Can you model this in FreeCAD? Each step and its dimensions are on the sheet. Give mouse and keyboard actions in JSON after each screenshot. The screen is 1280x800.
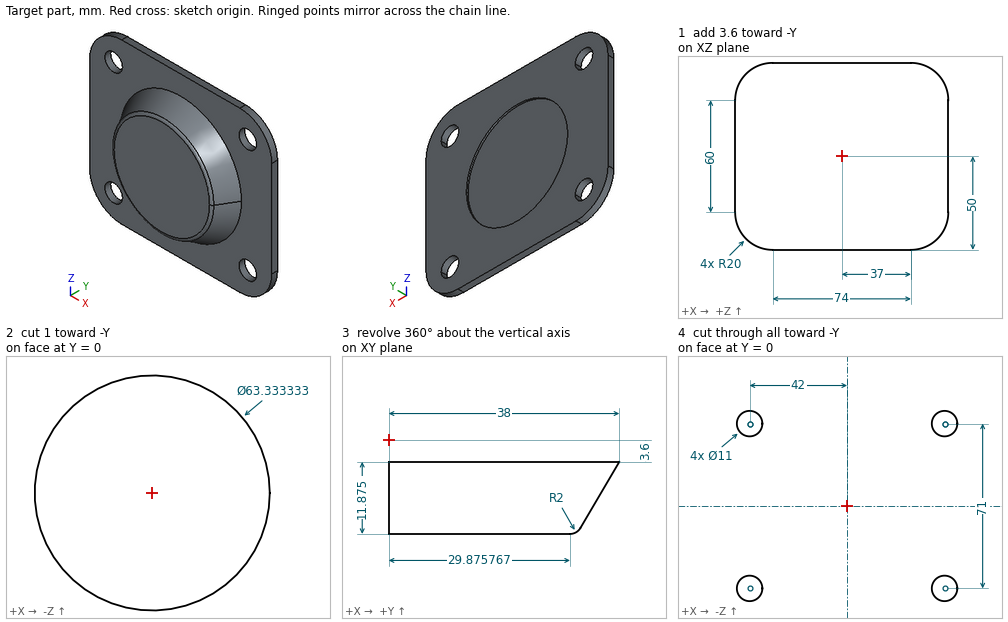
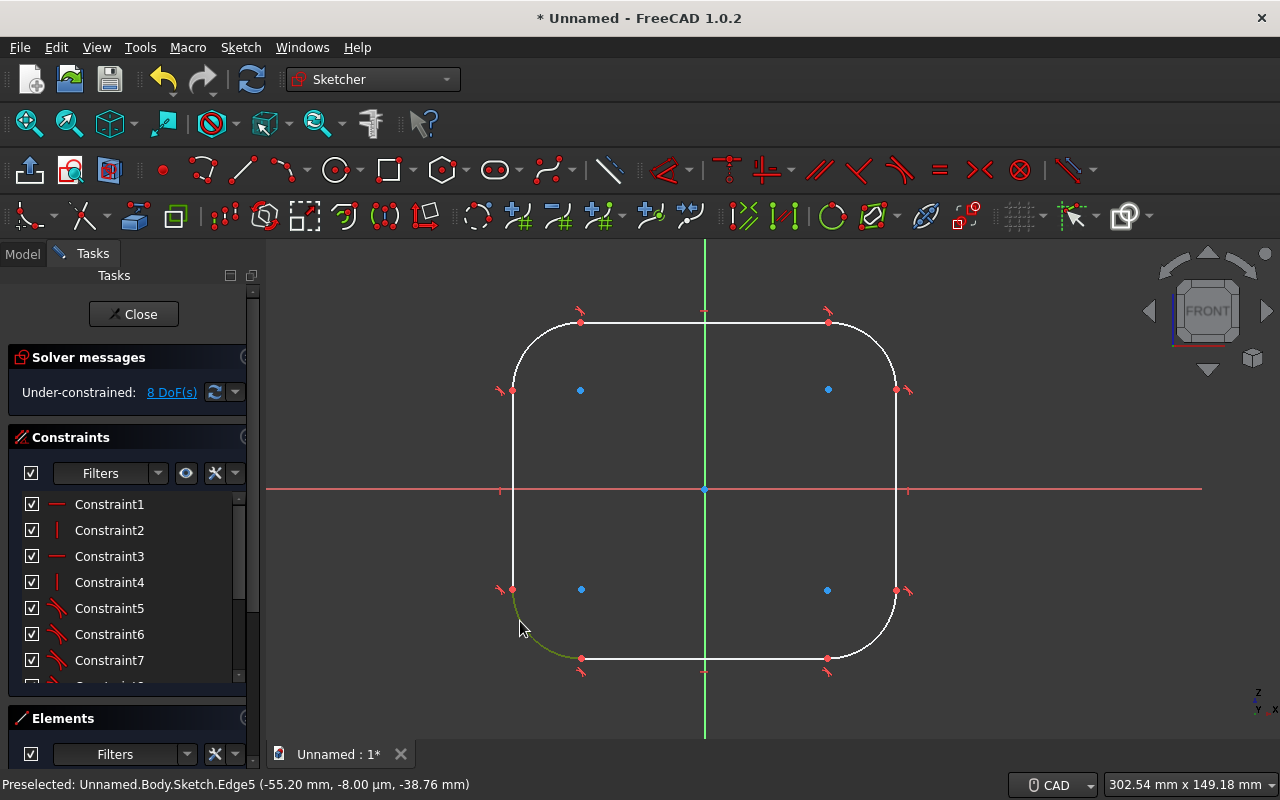
{"action": "left_click", "coordinate": [550, 330]}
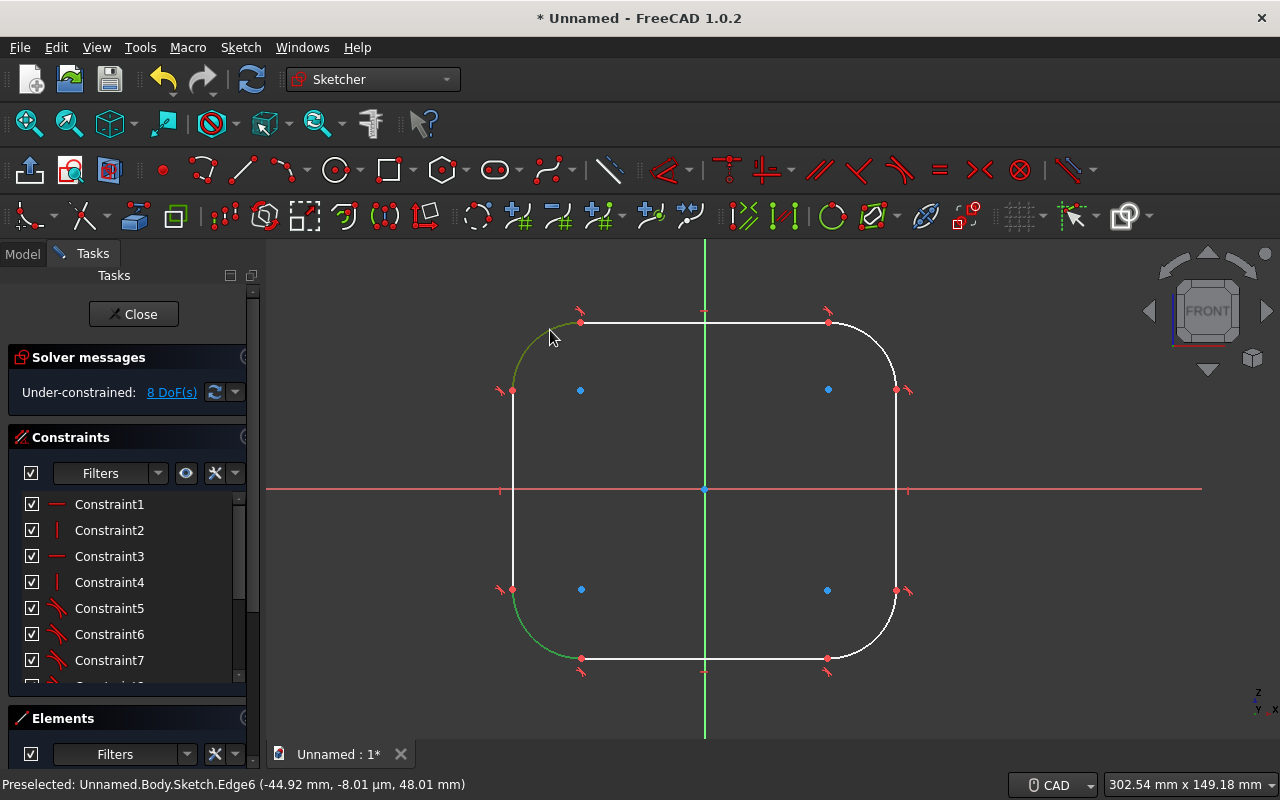
{"action": "left_click", "coordinate": [889, 359]}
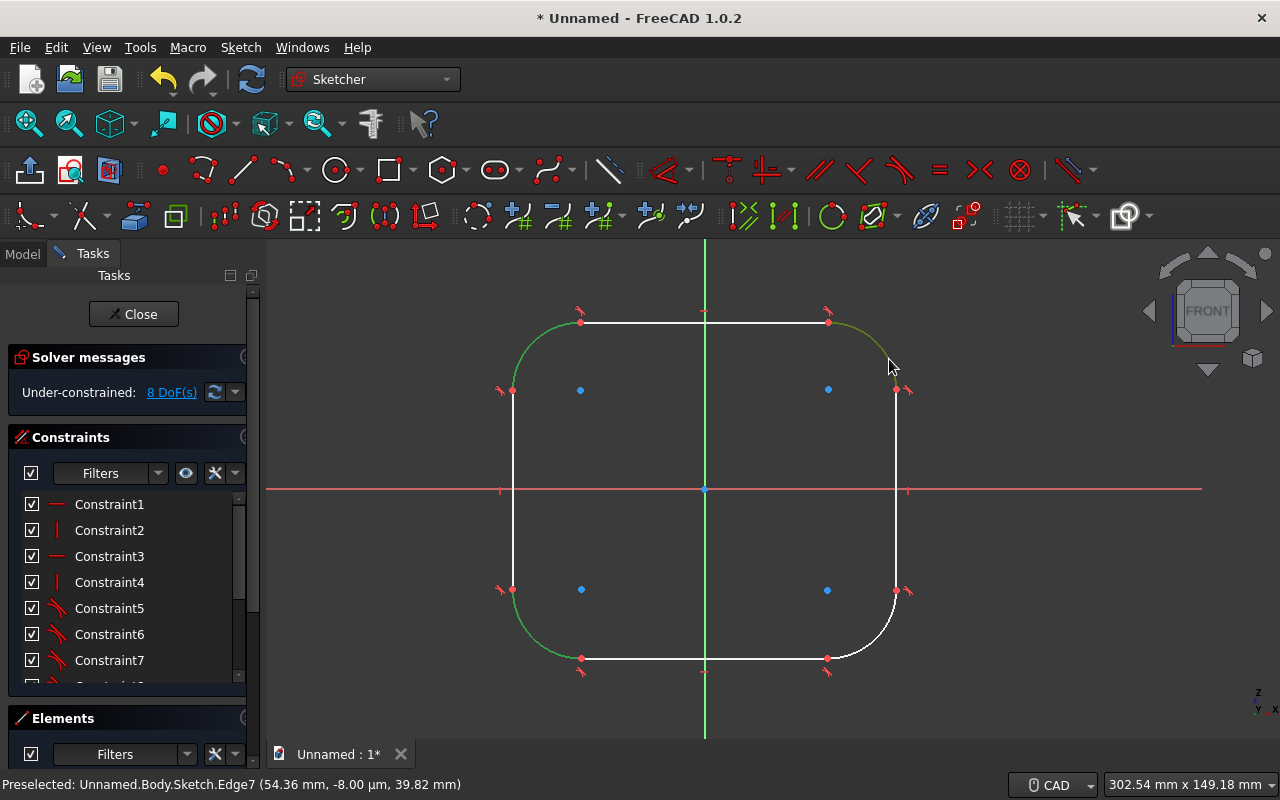
{"action": "left_click", "coordinate": [859, 651]}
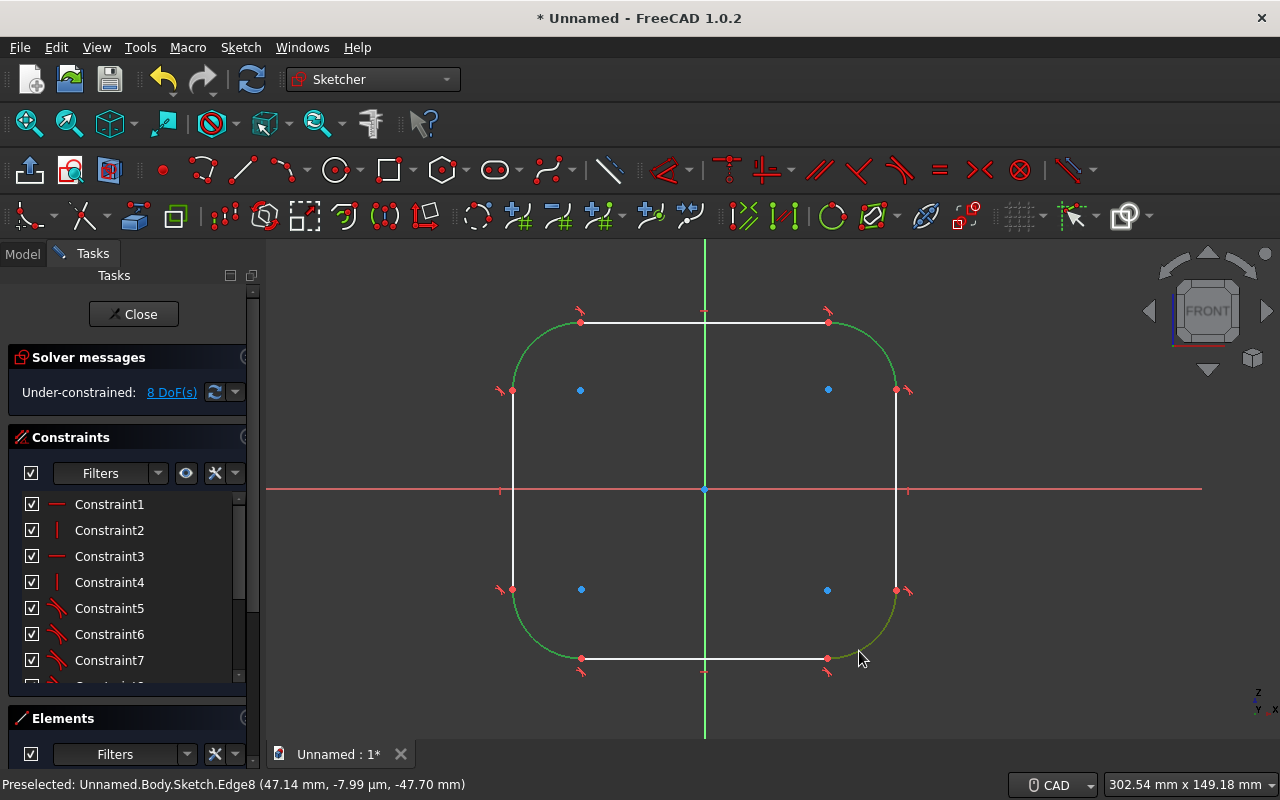
{"action": "left_click", "coordinate": [940, 170]}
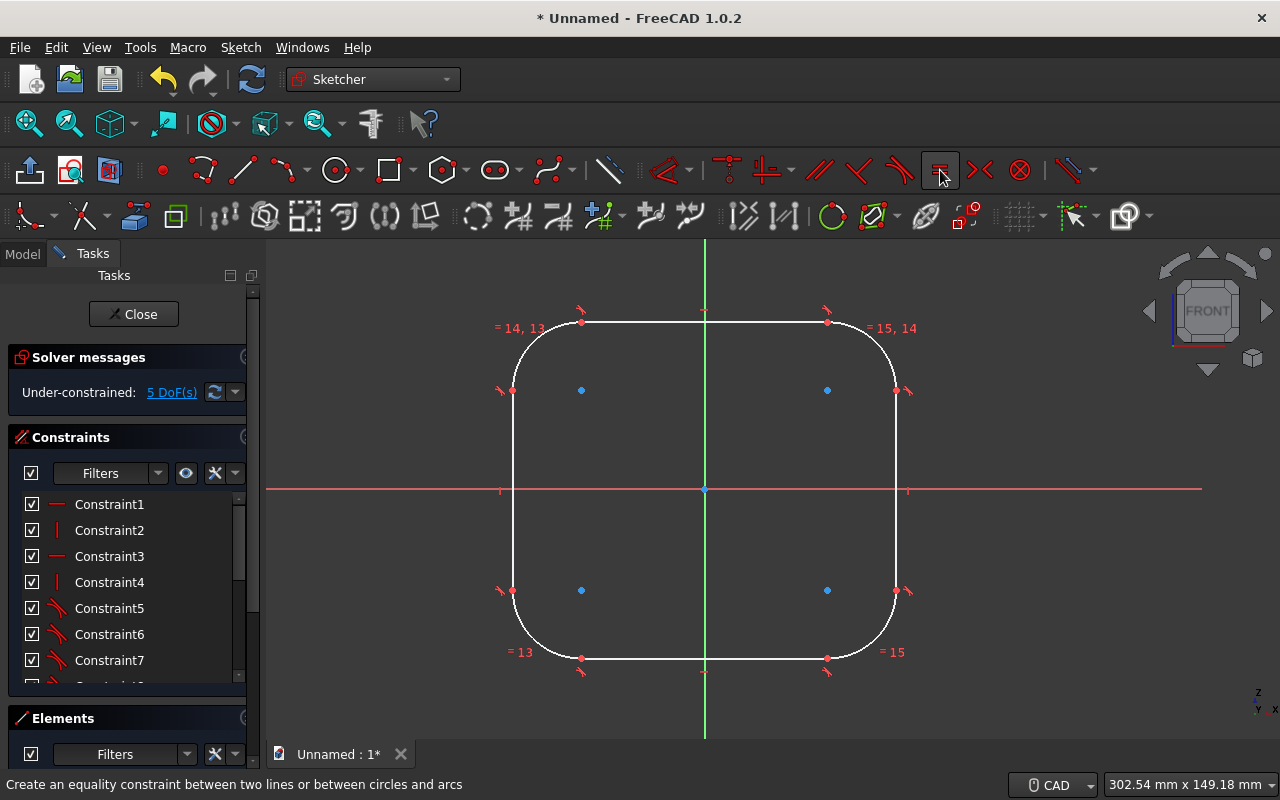
{"action": "left_click", "coordinate": [664, 170]}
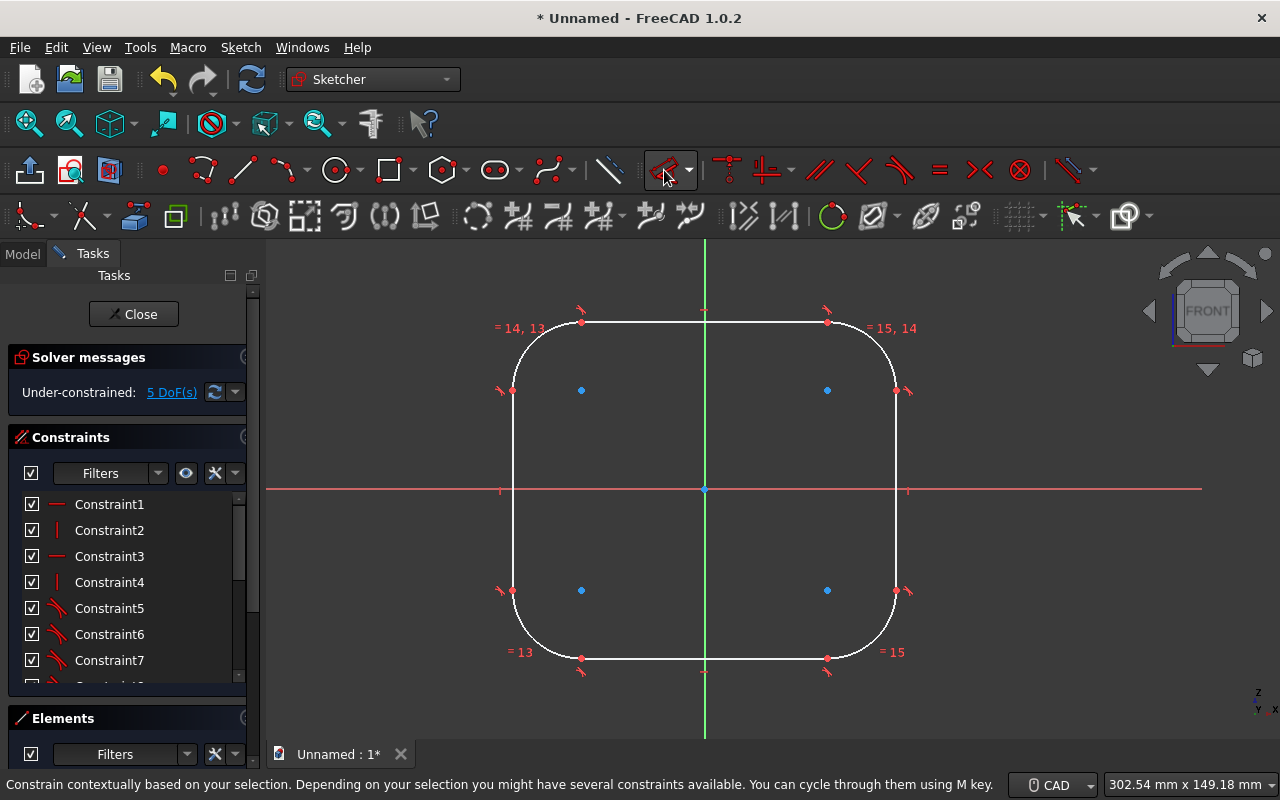
{"action": "left_click", "coordinate": [520, 621]}
{"action": "left_click", "coordinate": [491, 635]}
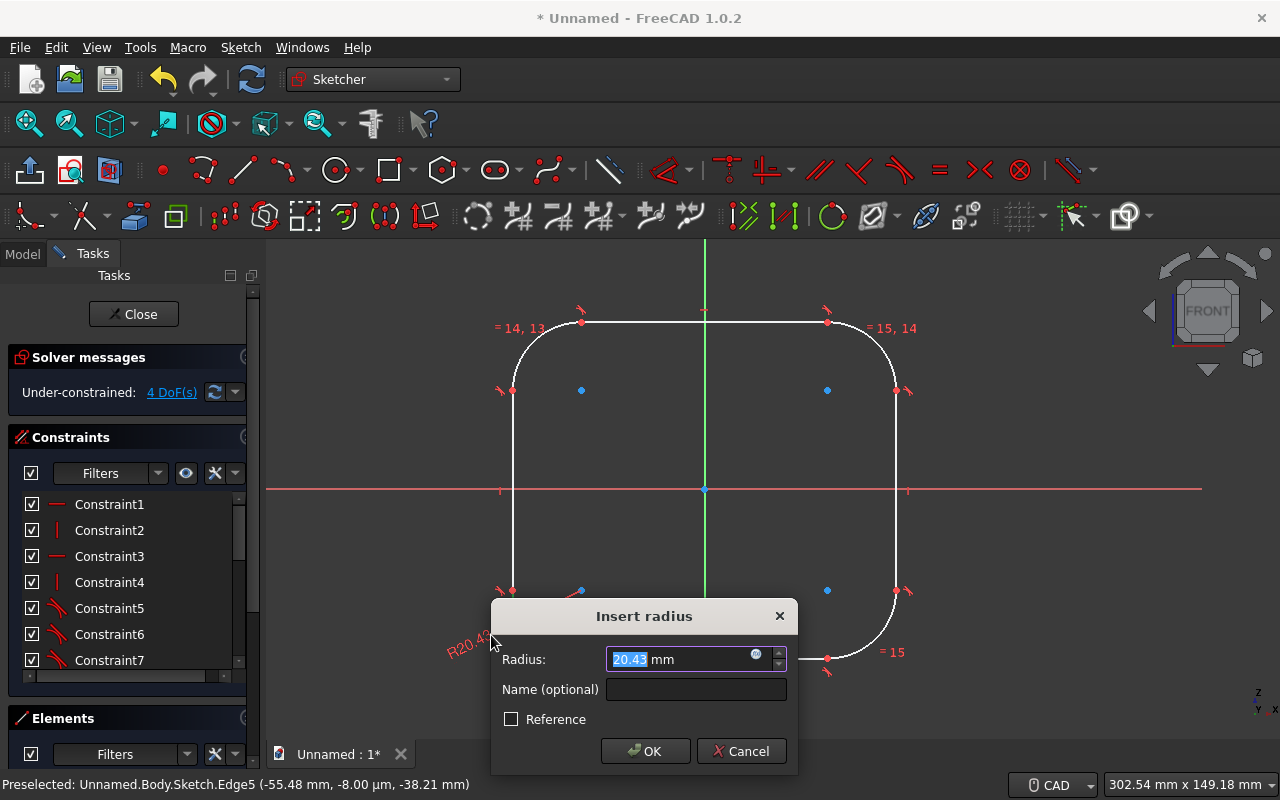
{"action": "type", "text": "20"}
{"action": "key", "text": "Return"}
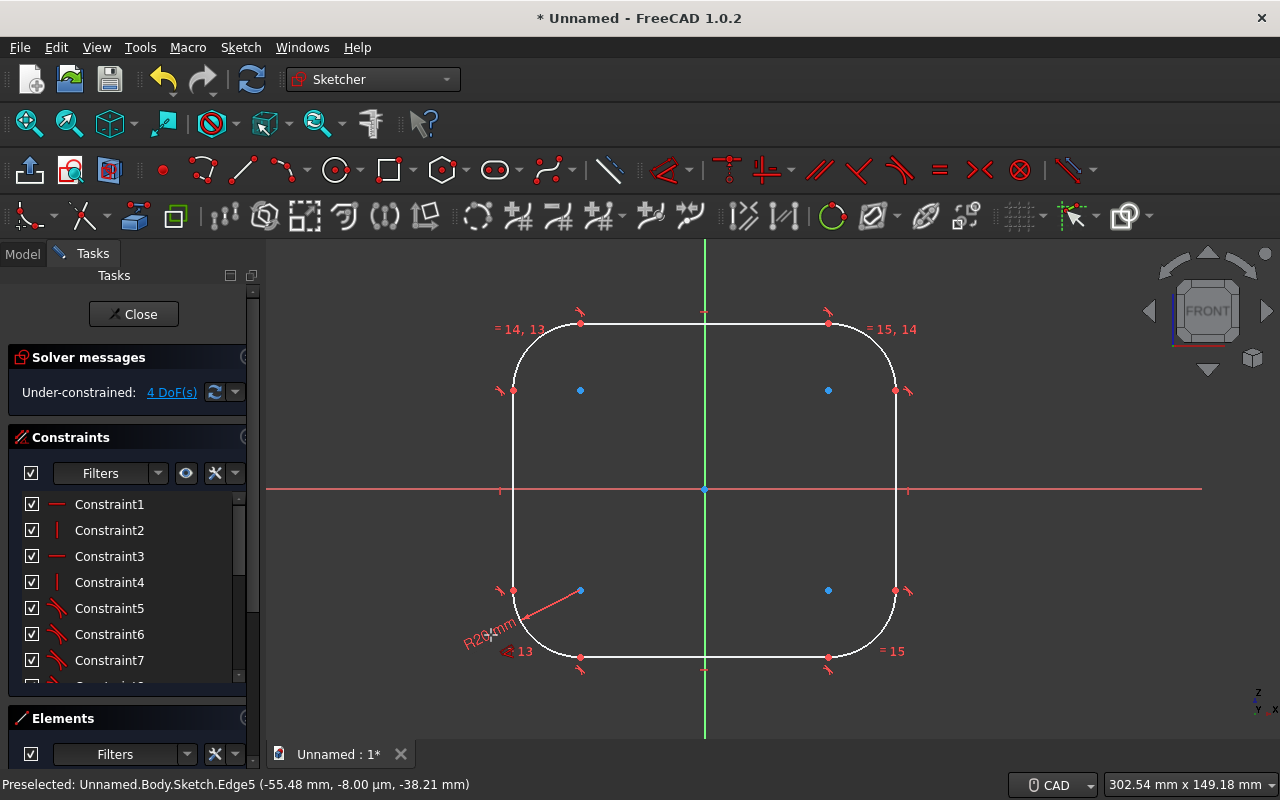
{"action": "left_click", "coordinate": [754, 657]}
{"action": "left_click", "coordinate": [647, 691]}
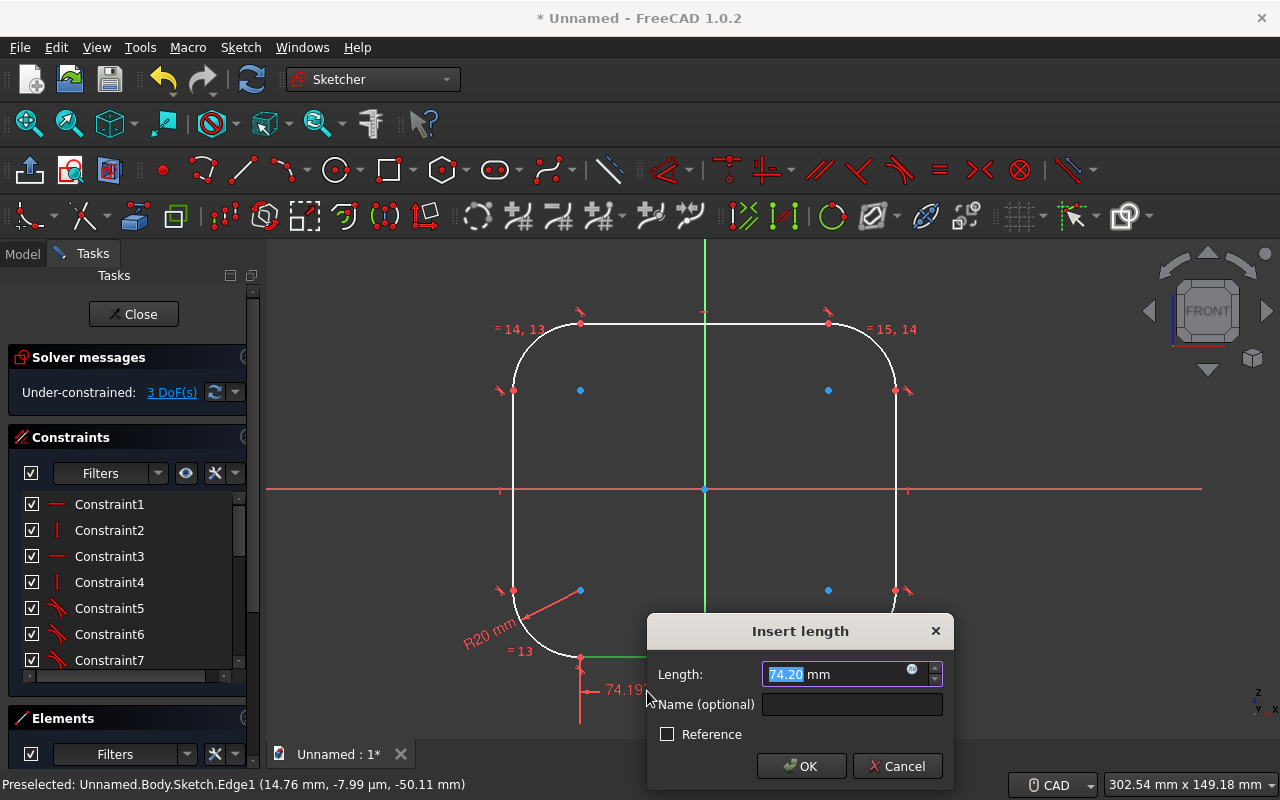
{"action": "type", "text": "74"}
{"action": "key", "text": "Return"}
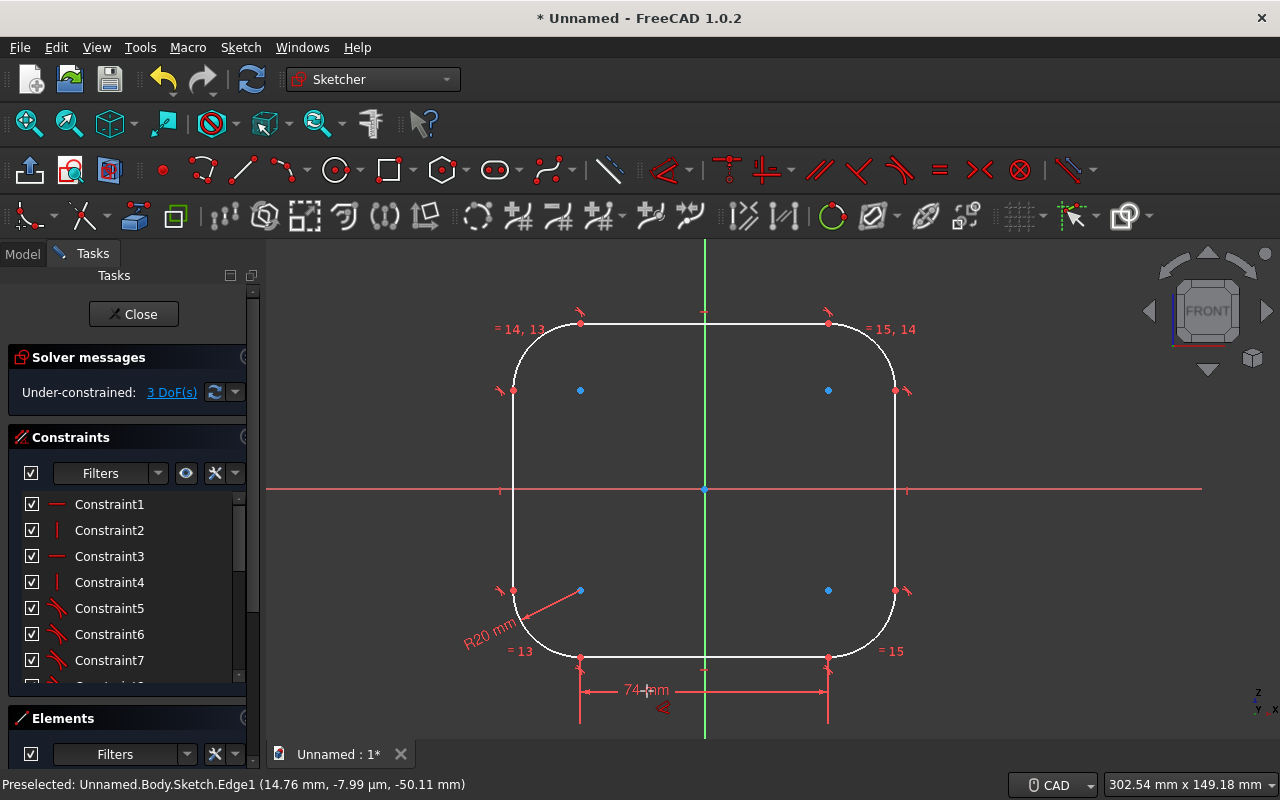
{"action": "left_click", "coordinate": [513, 530]}
{"action": "left_click", "coordinate": [479, 445]}